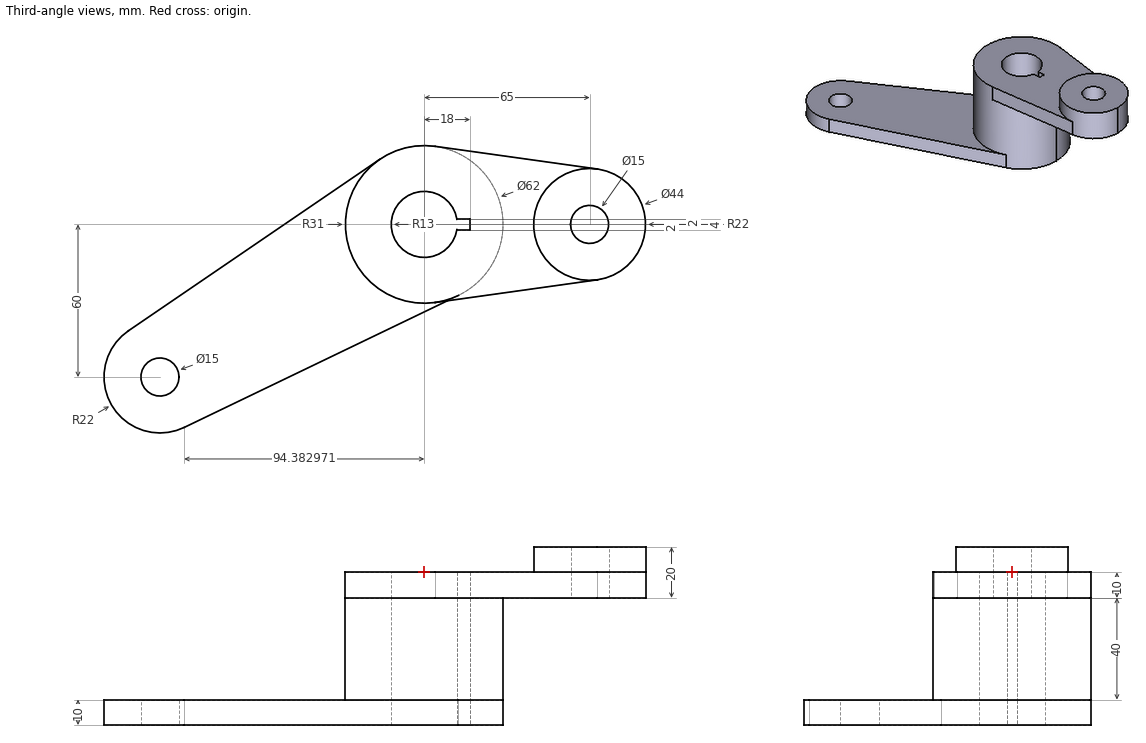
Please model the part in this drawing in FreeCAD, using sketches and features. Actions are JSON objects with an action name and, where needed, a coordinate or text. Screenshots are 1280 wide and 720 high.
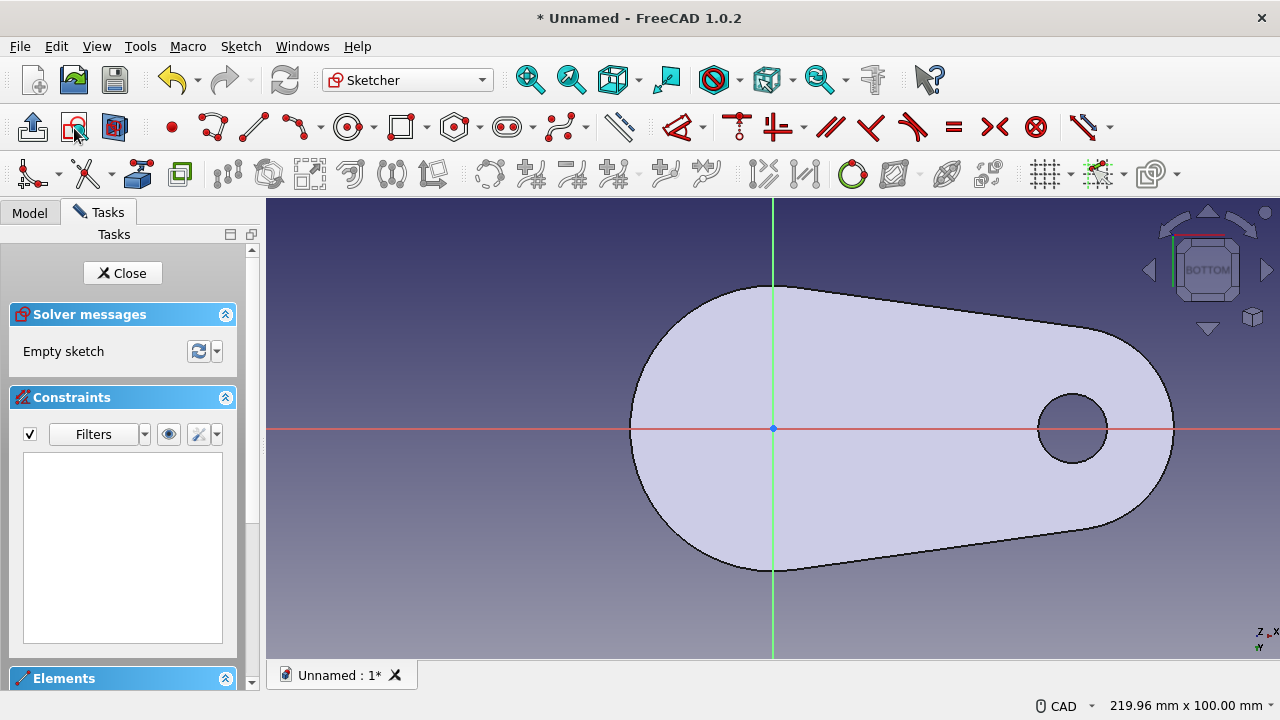
{"action": "scroll", "coordinate": [832, 419], "scroll_direction": "up", "scroll_amount": 3}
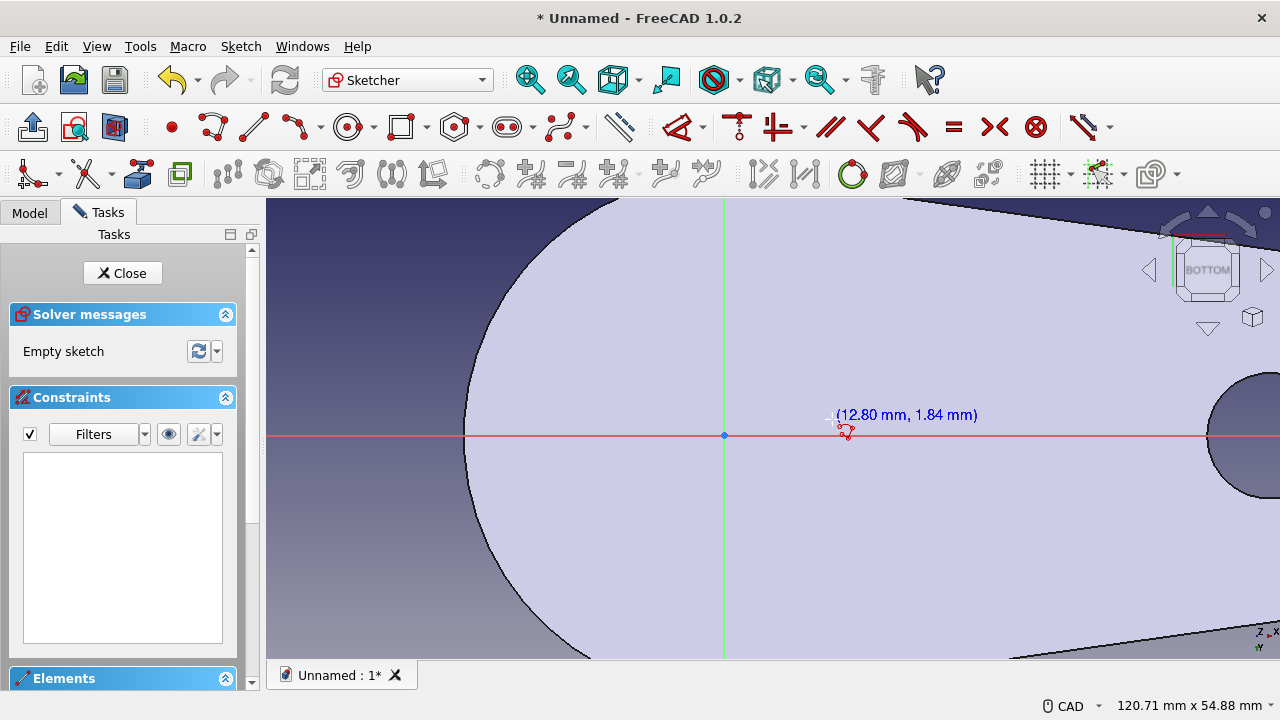
{"action": "left_click", "coordinate": [832, 419]}
{"action": "left_click", "coordinate": [875, 419]}
{"action": "left_click", "coordinate": [875, 453]}
{"action": "left_click", "coordinate": [832, 453]}
{"action": "right_click", "coordinate": [832, 453]}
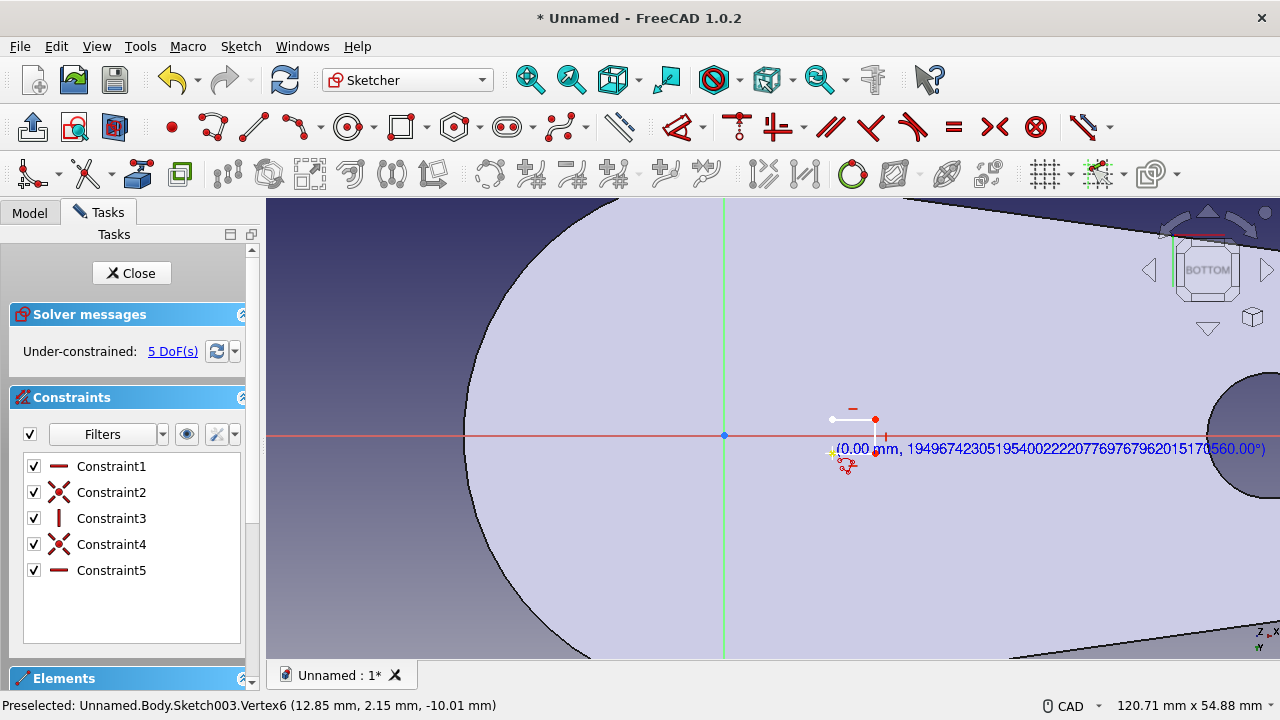
{"action": "key", "text": "g 3 a"}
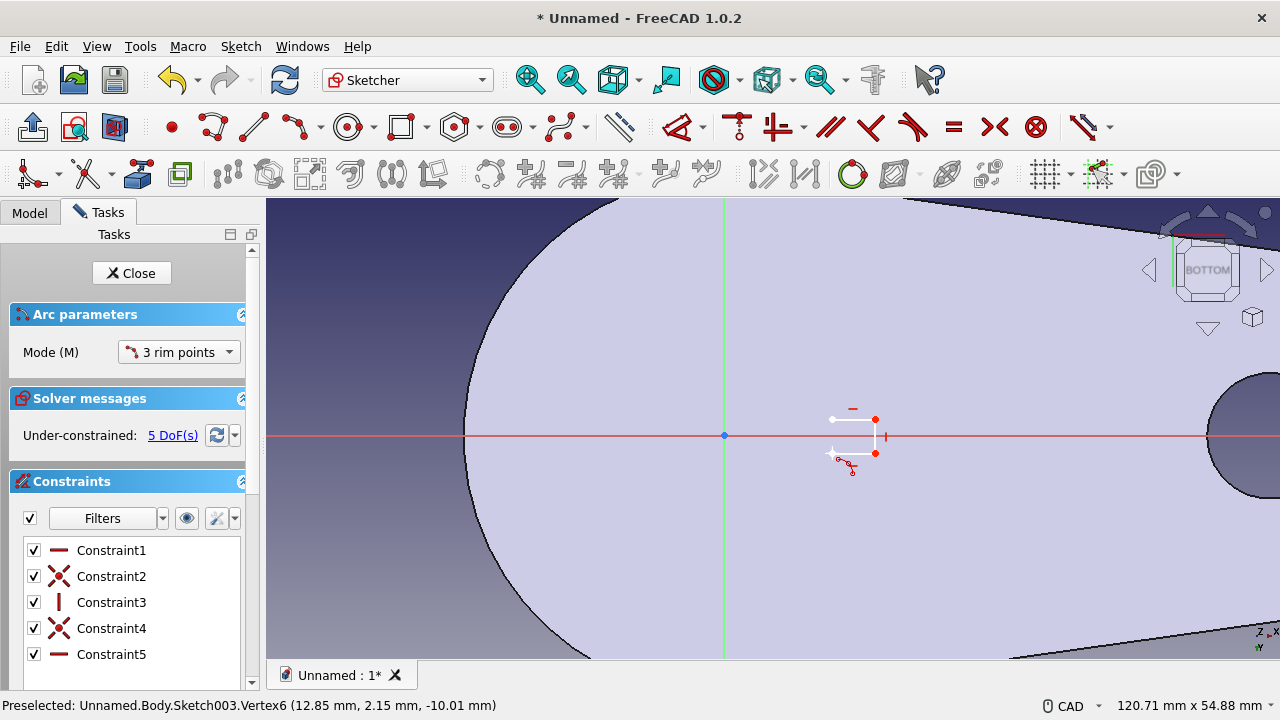
{"action": "left_click", "coordinate": [832, 454]}
{"action": "left_click", "coordinate": [832, 420]}
{"action": "left_click", "coordinate": [634, 374]}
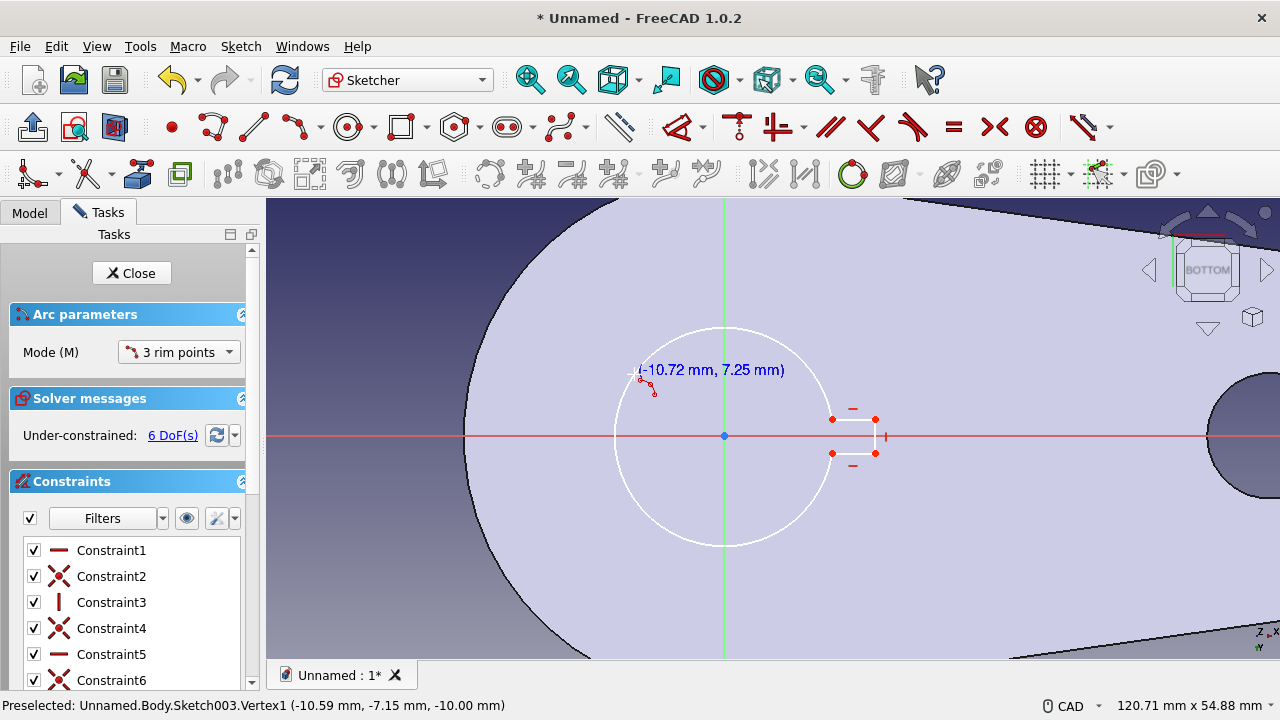
{"action": "key", "text": "g c"}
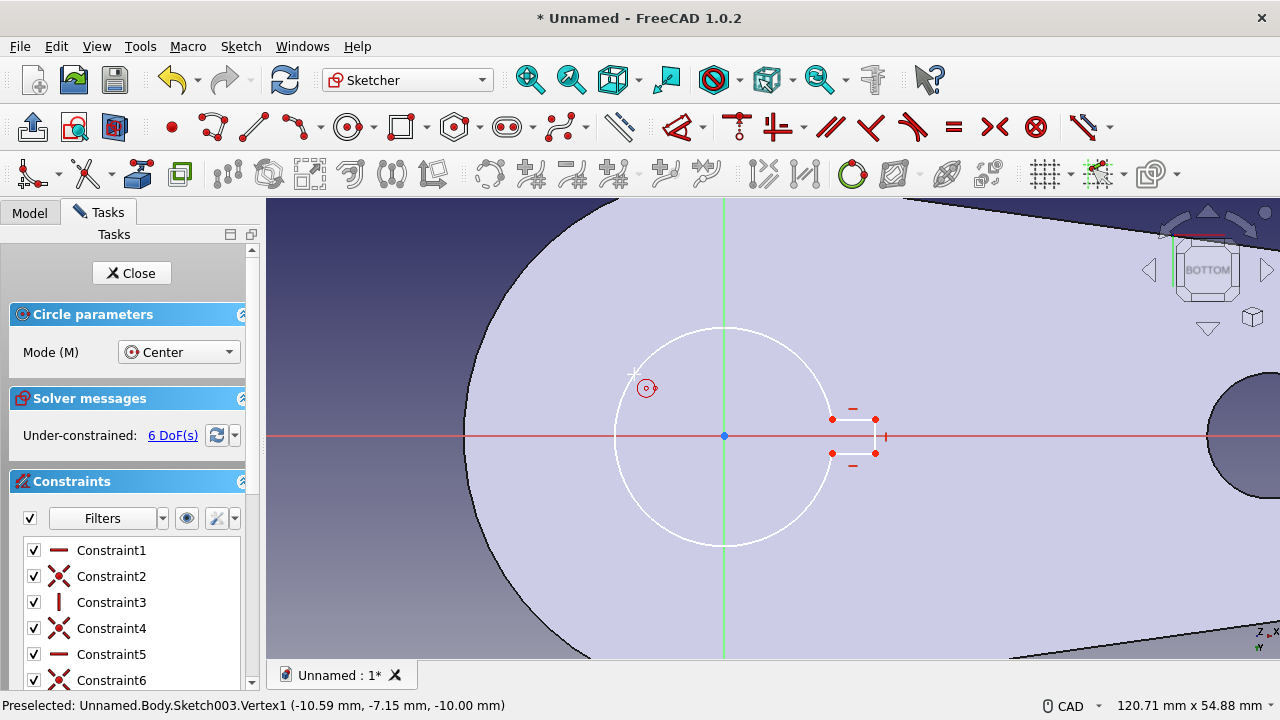
{"action": "left_click", "coordinate": [724, 436]}
{"action": "left_click", "coordinate": [908, 252]}
{"action": "key", "text": "Escape"}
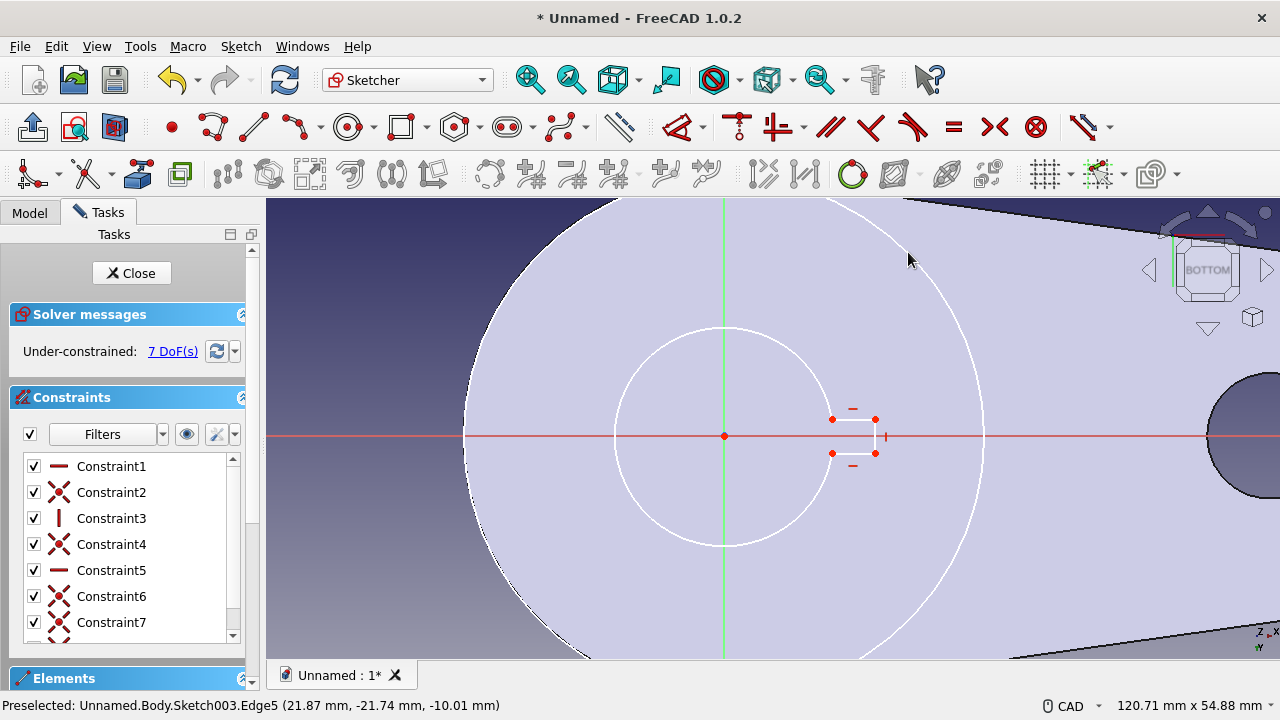
{"action": "left_click_drag", "start_coordinate": [714, 426], "coordinate": [734, 447]}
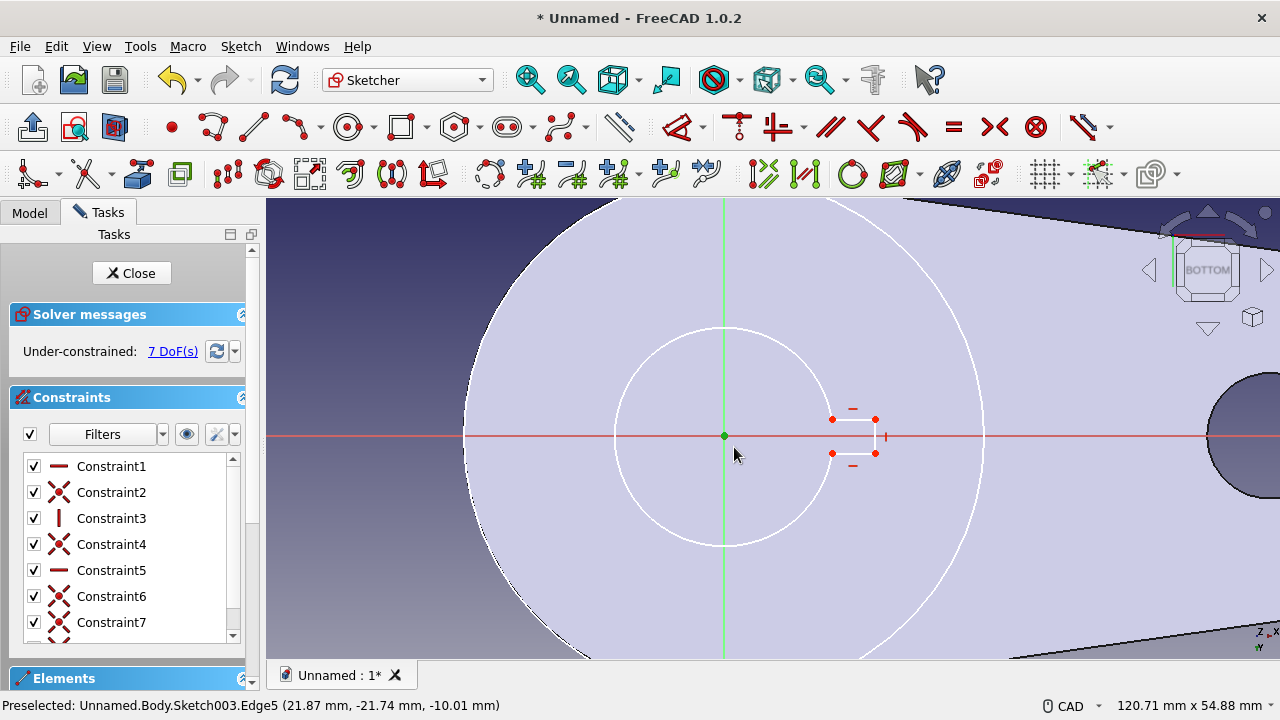
{"action": "key", "text": "c"}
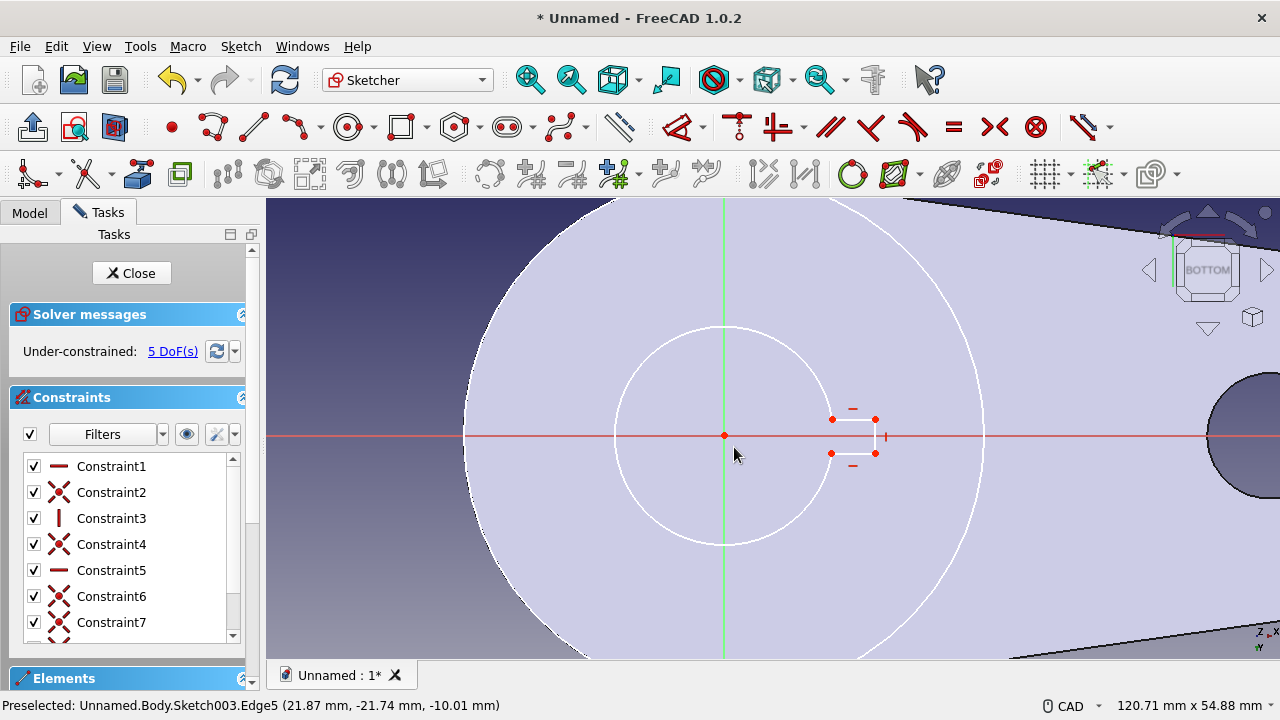
{"action": "left_click", "coordinate": [676, 128]}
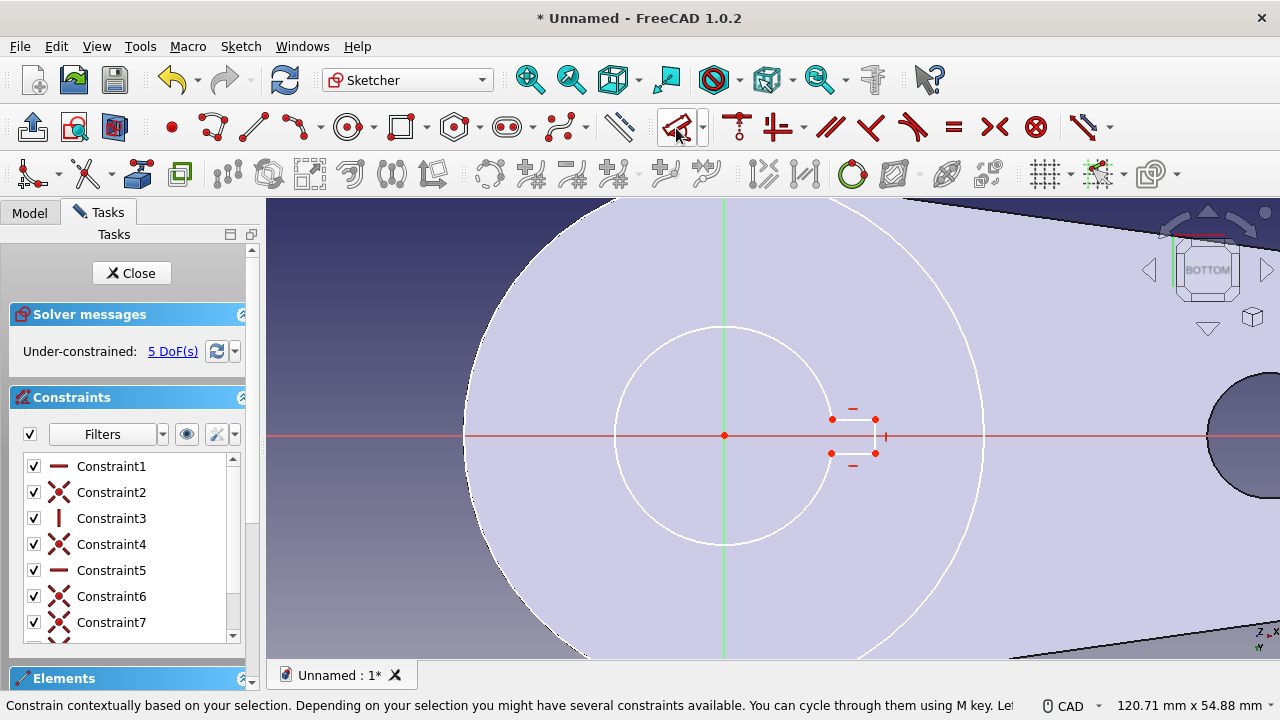
{"action": "left_click", "coordinate": [685, 334]}
{"action": "left_click", "coordinate": [674, 304]}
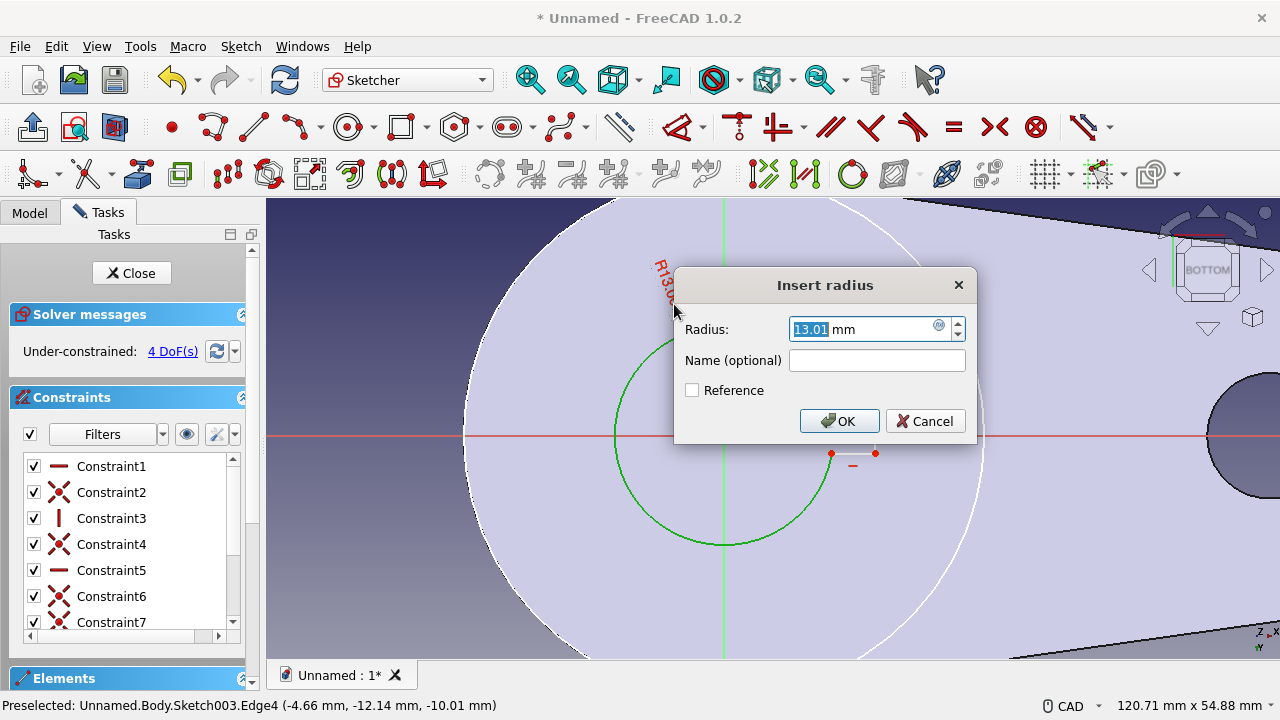
{"action": "type", "text": "13"}
{"action": "key", "text": "Return"}